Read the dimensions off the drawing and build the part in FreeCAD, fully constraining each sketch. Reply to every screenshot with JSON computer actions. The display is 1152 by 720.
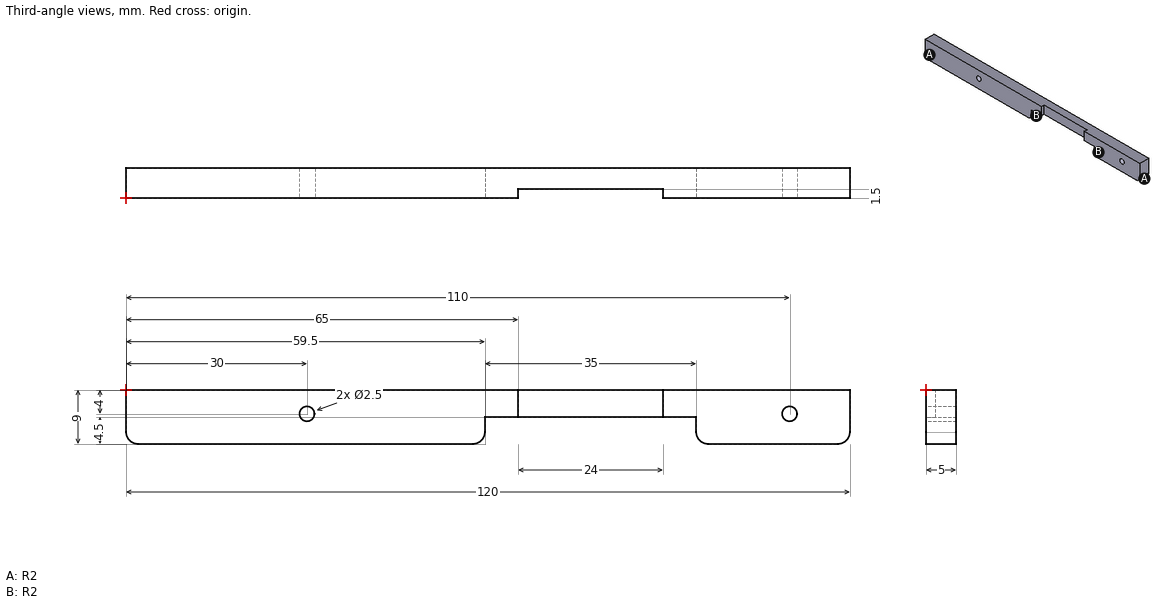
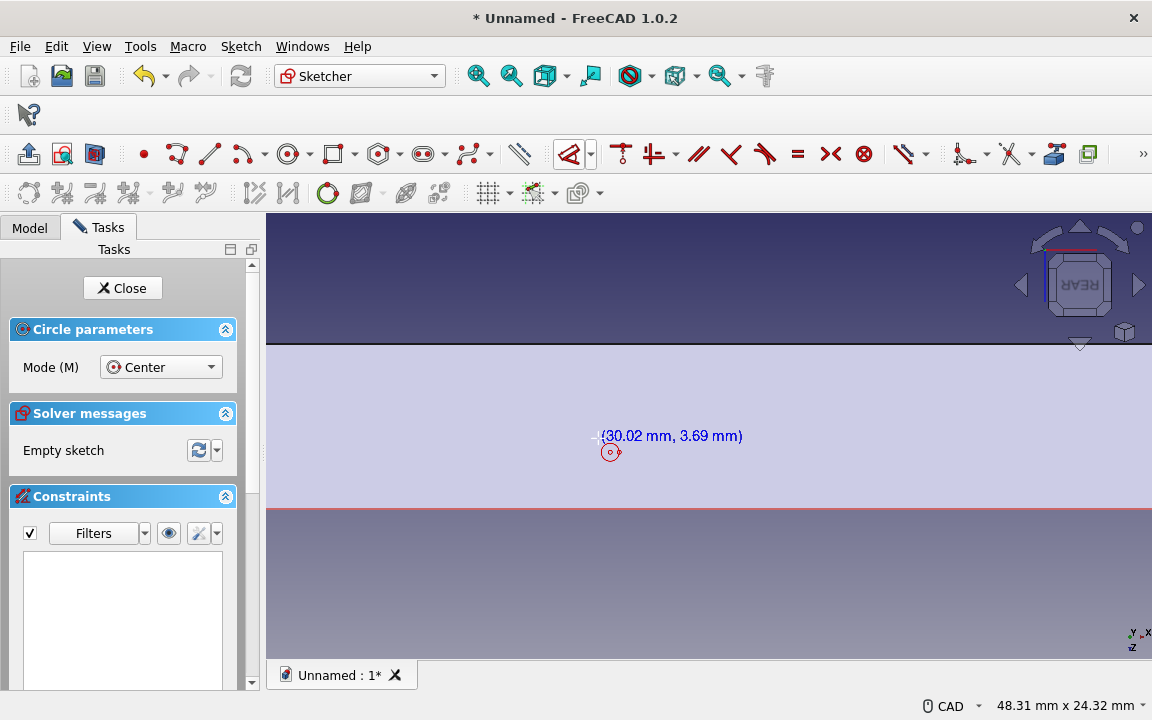
{"action": "scroll", "coordinate": [501, 428], "scroll_direction": "down", "scroll_amount": 7}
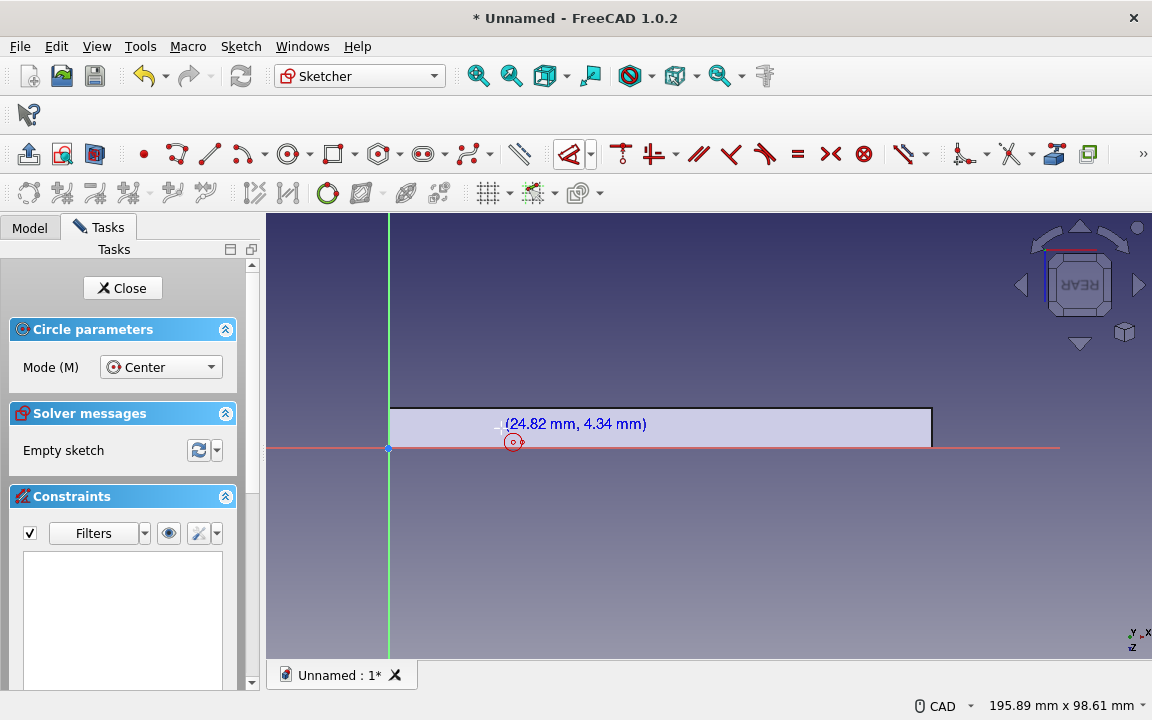
{"action": "left_click", "coordinate": [525, 430]}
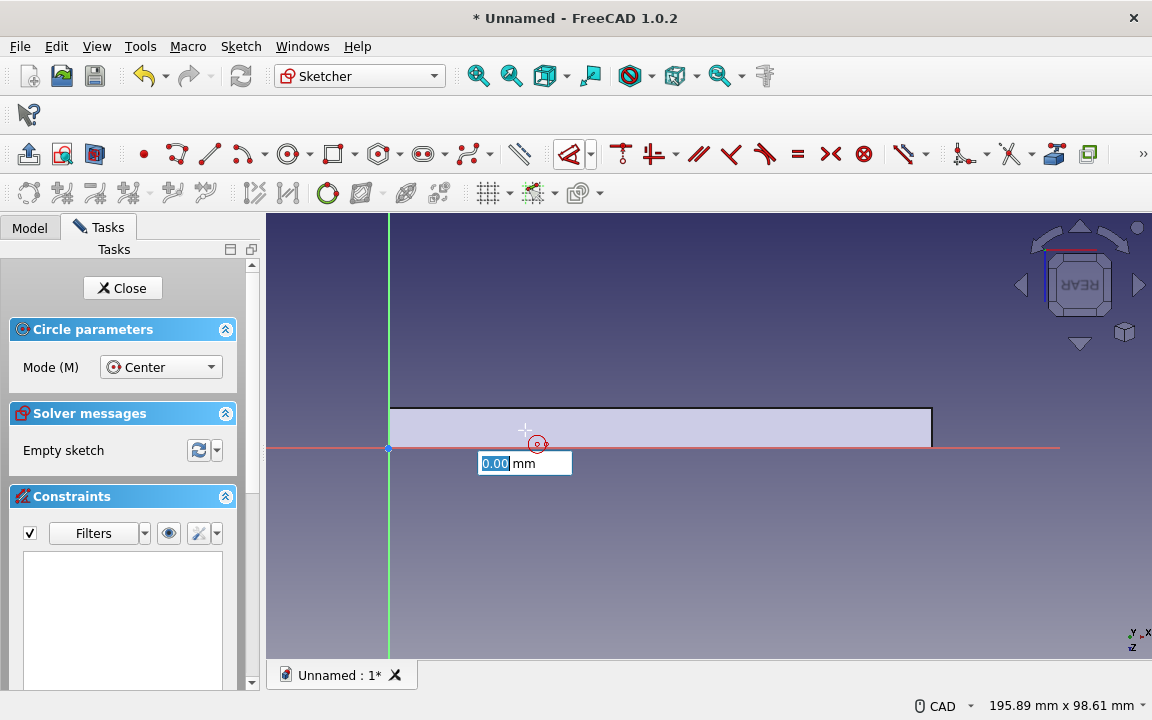
{"action": "scroll", "coordinate": [529, 426], "scroll_direction": "up", "scroll_amount": 6}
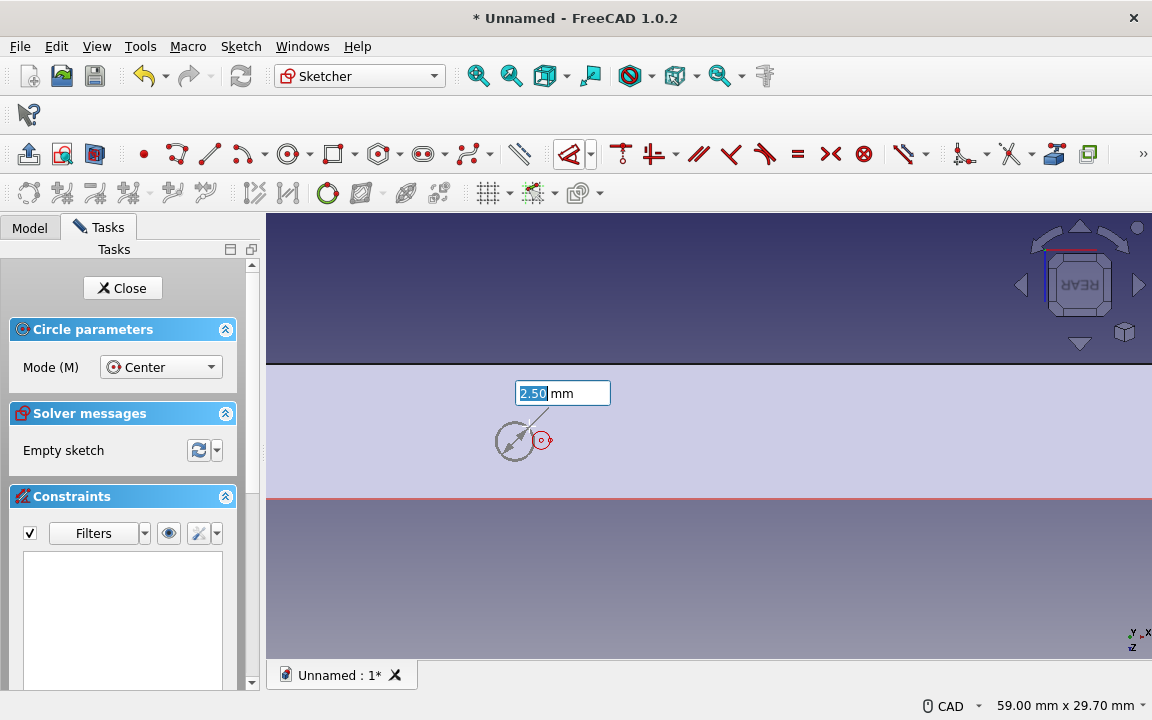
{"action": "left_click", "coordinate": [527, 425]}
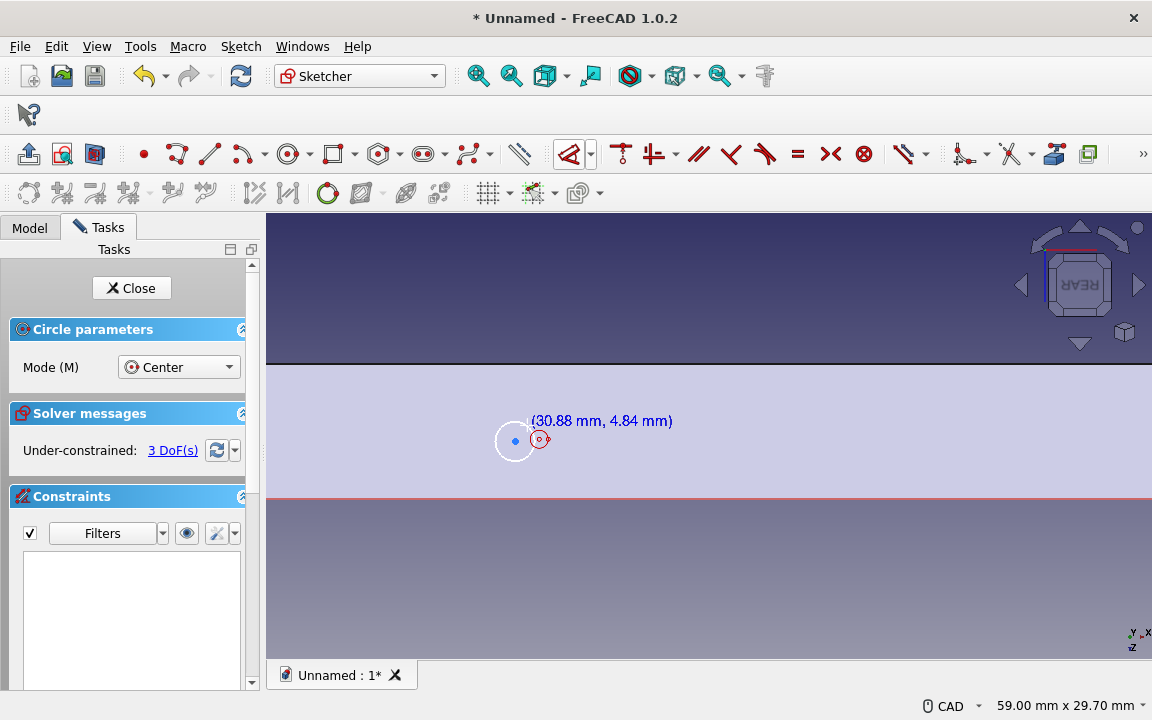
{"action": "scroll", "coordinate": [529, 426], "scroll_direction": "down", "scroll_amount": 6}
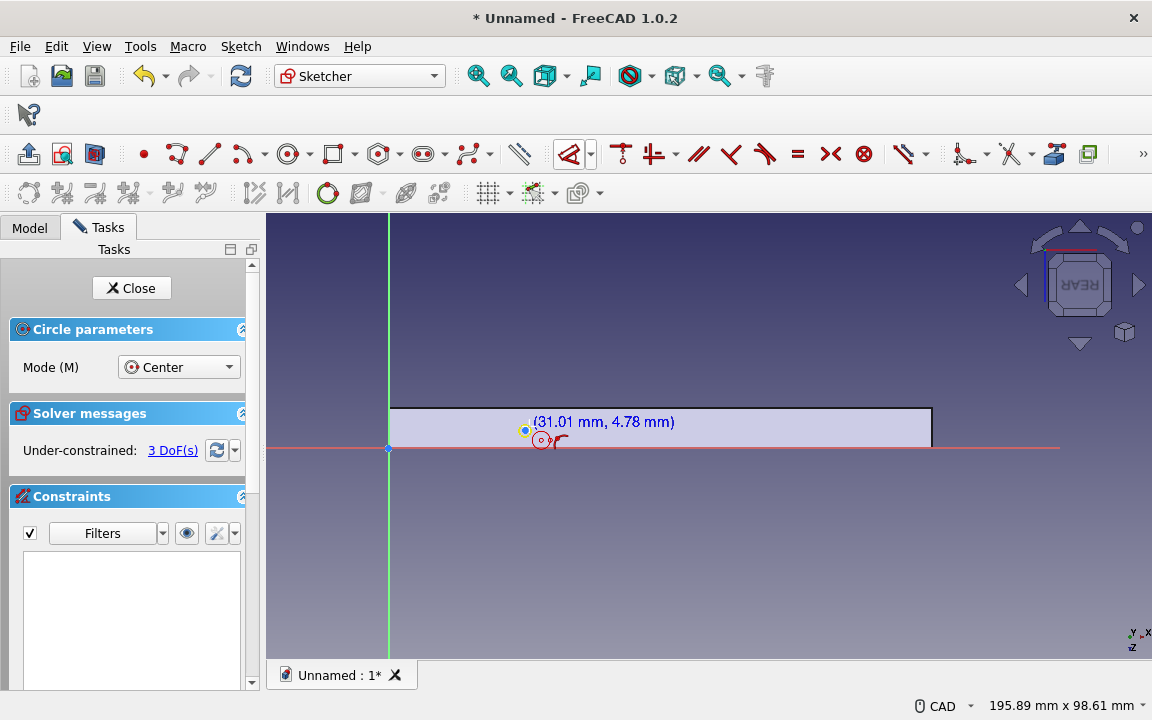
{"action": "scroll", "coordinate": [886, 430], "scroll_direction": "up", "scroll_amount": 7}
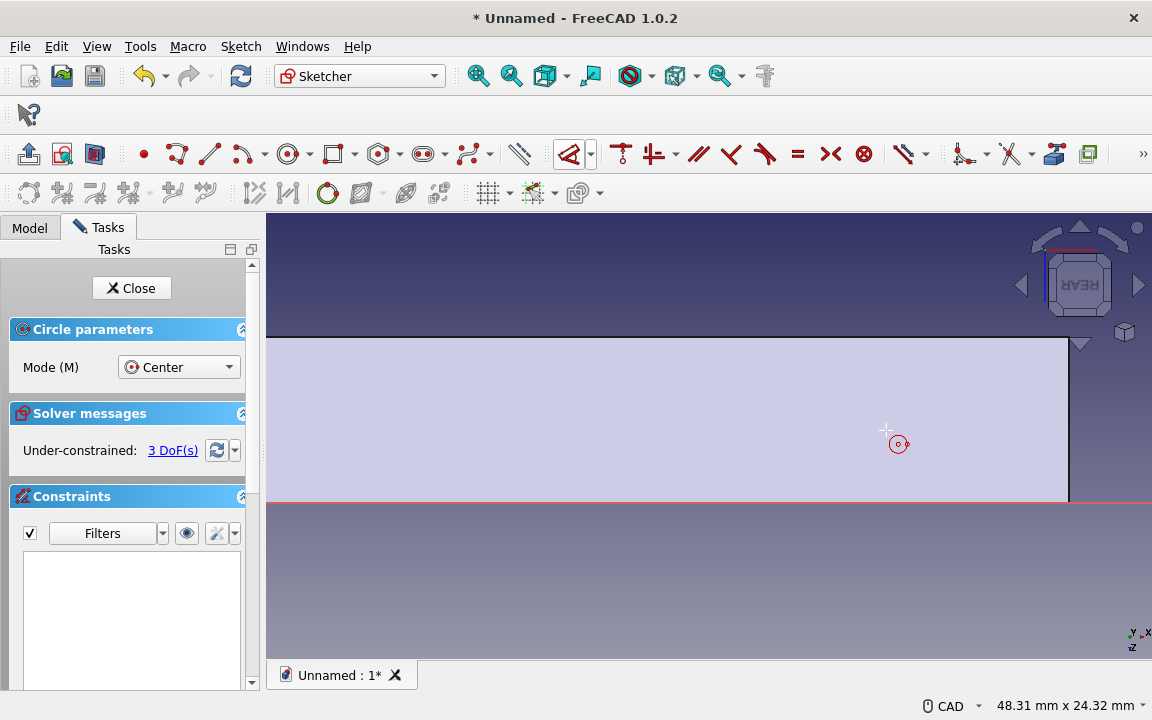
{"action": "scroll", "coordinate": [887, 430], "scroll_direction": "down", "scroll_amount": 7}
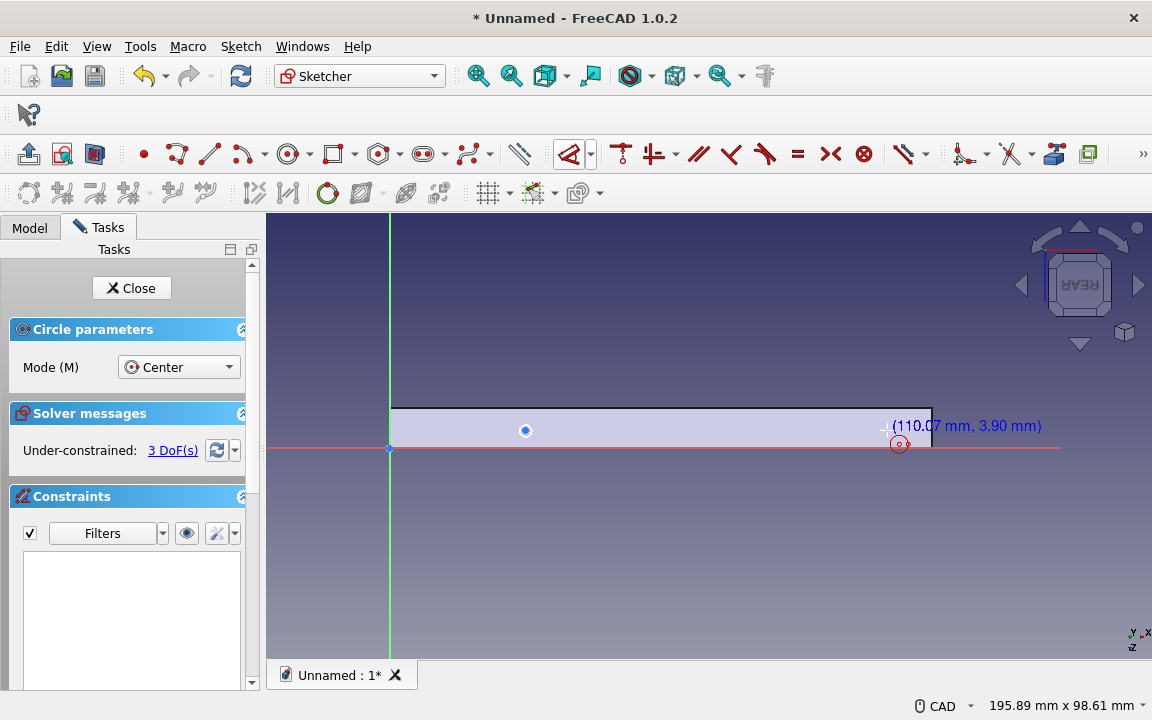
{"action": "left_click", "coordinate": [887, 430]}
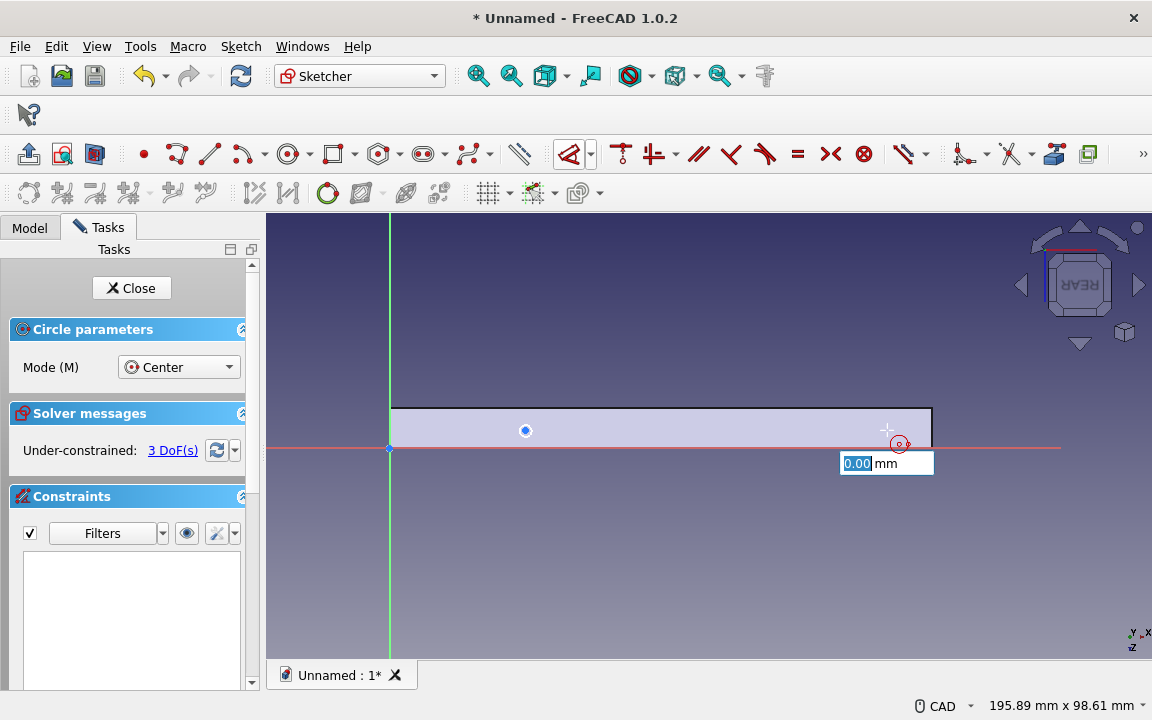
{"action": "scroll", "coordinate": [891, 426], "scroll_direction": "up", "scroll_amount": 6}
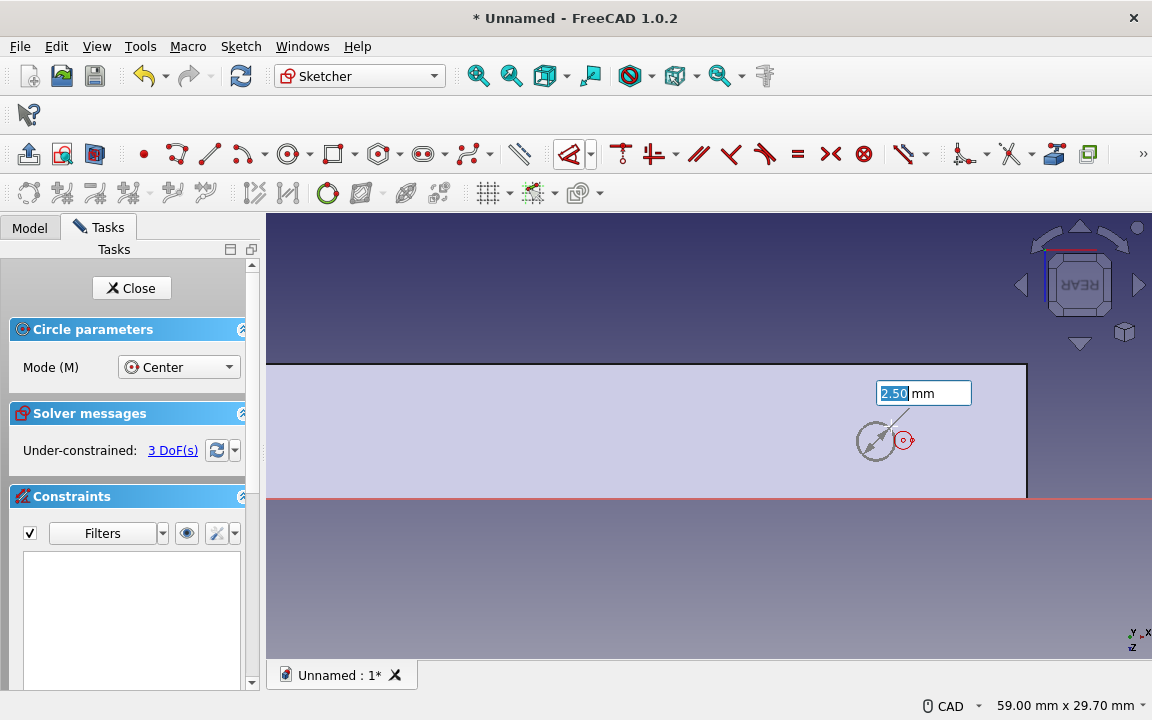
{"action": "left_click", "coordinate": [890, 425]}
{"action": "key", "text": "Escape"}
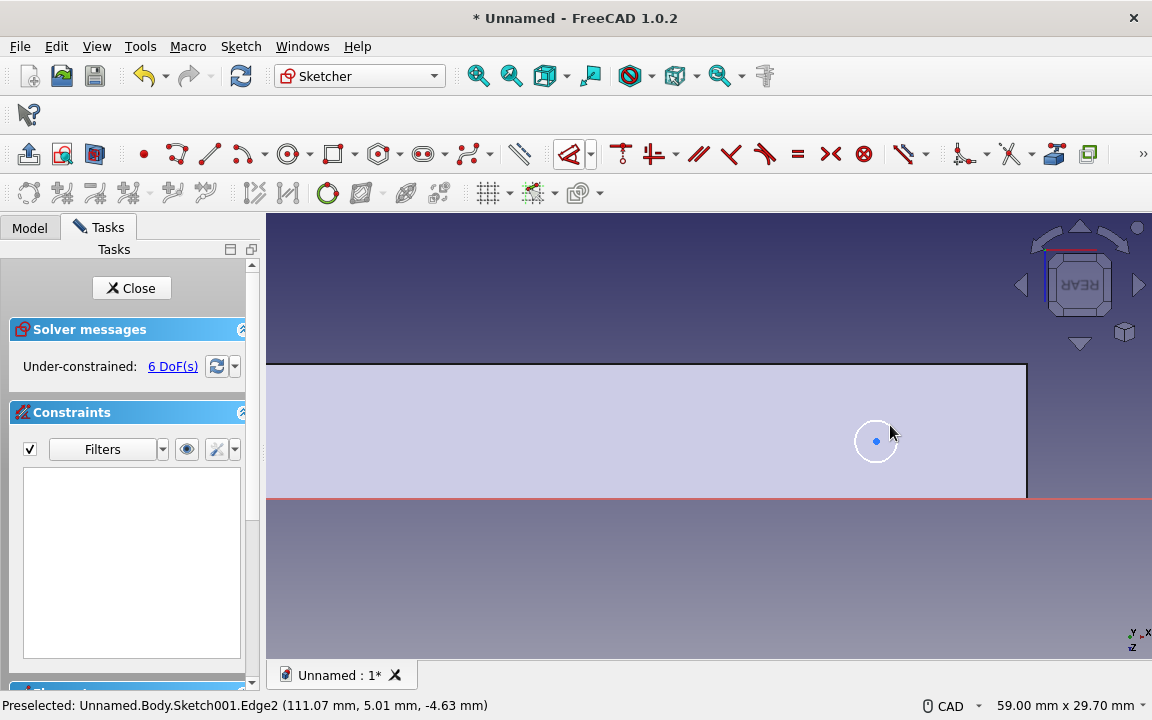
{"action": "scroll", "coordinate": [891, 426], "scroll_direction": "down", "scroll_amount": 6}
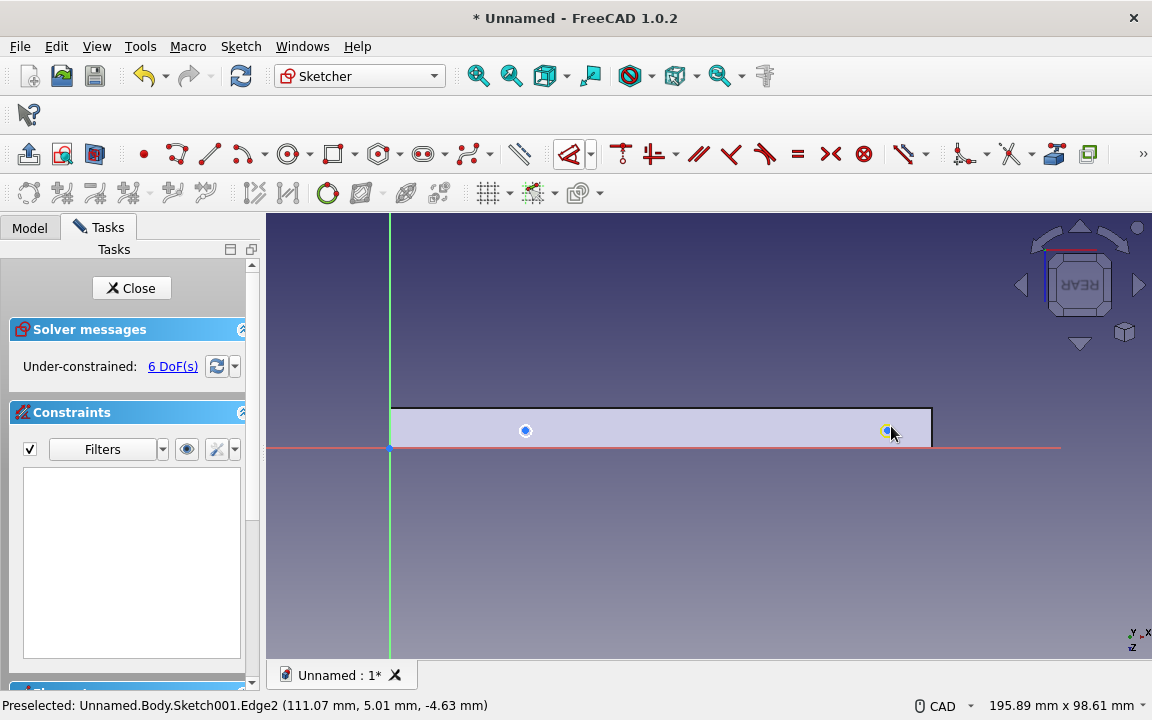
{"action": "scroll", "coordinate": [530, 427], "scroll_direction": "up", "scroll_amount": 5}